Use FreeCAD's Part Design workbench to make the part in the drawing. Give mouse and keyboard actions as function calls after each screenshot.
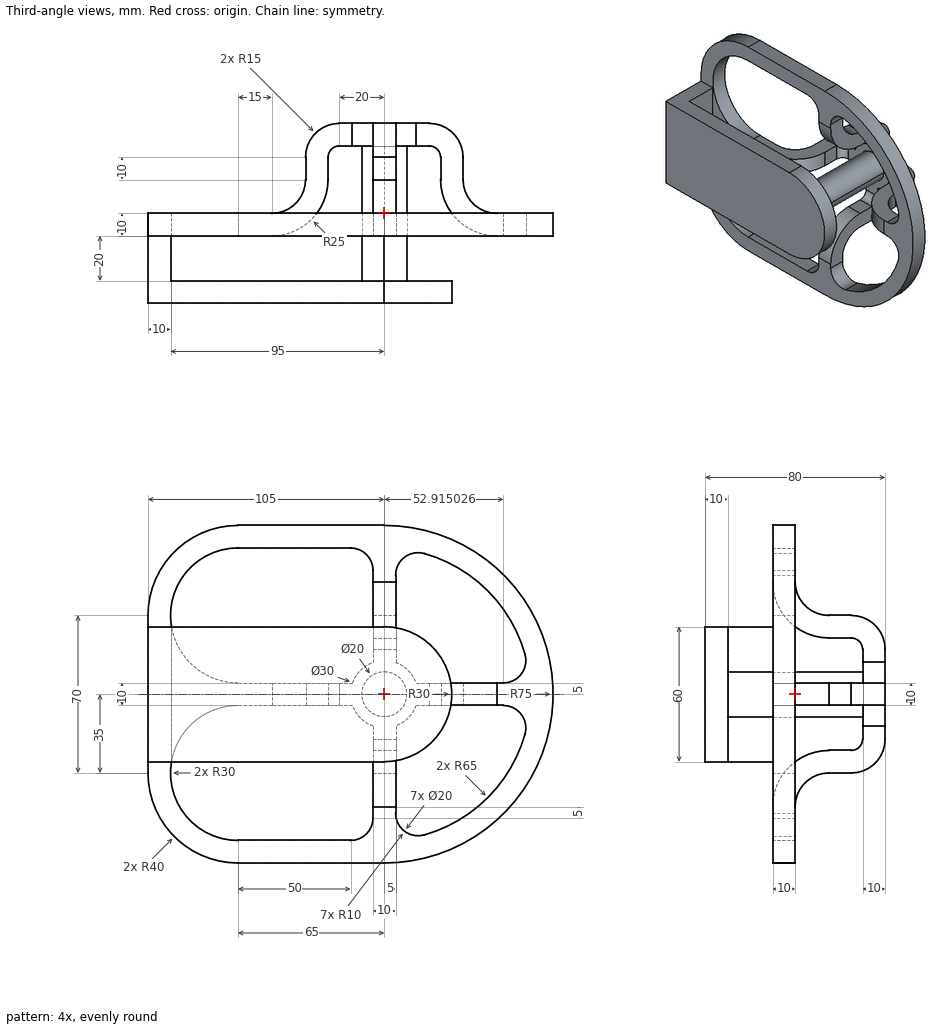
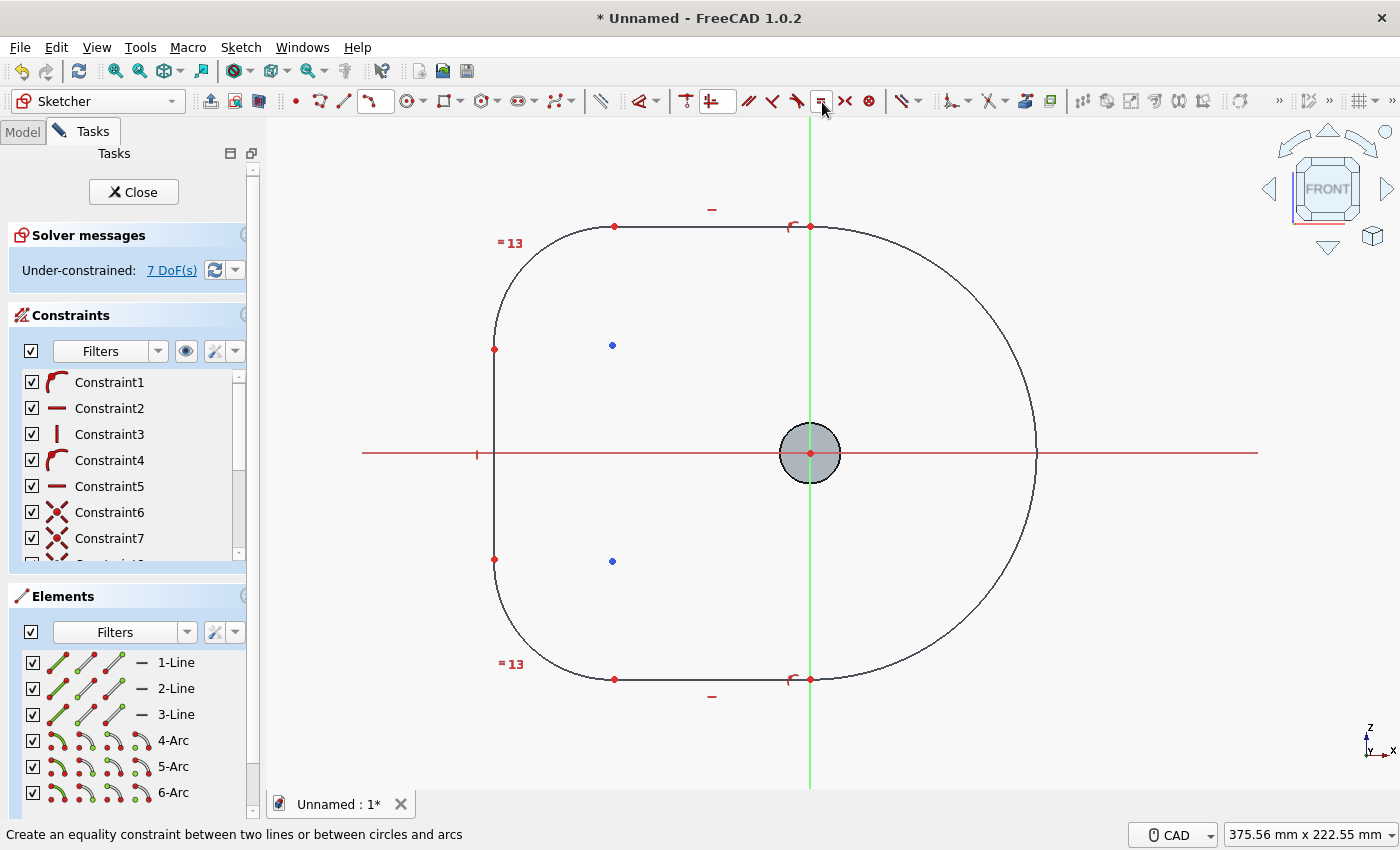
click(507, 615)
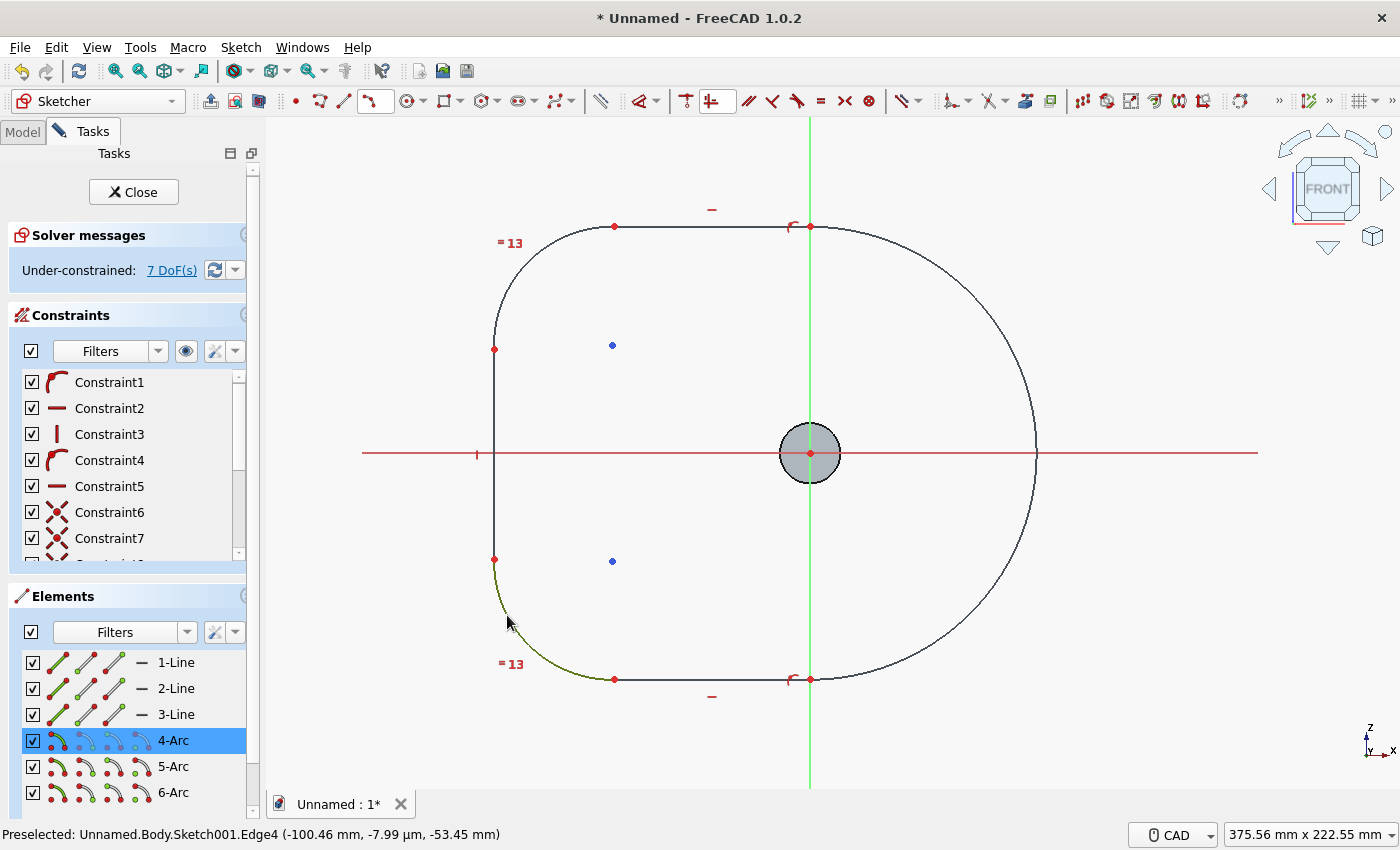
key(k)
key(r)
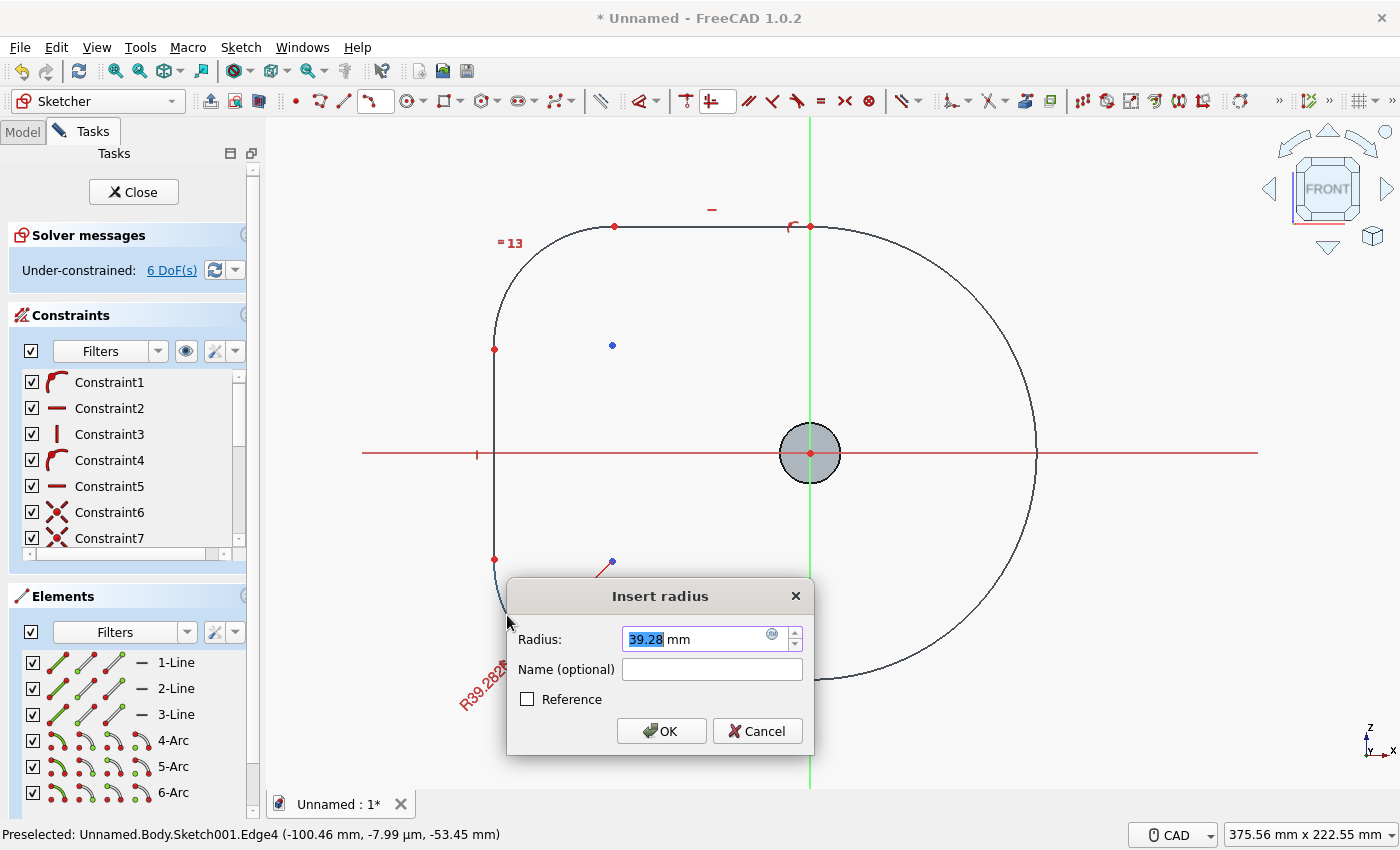
text(40)
key(Return)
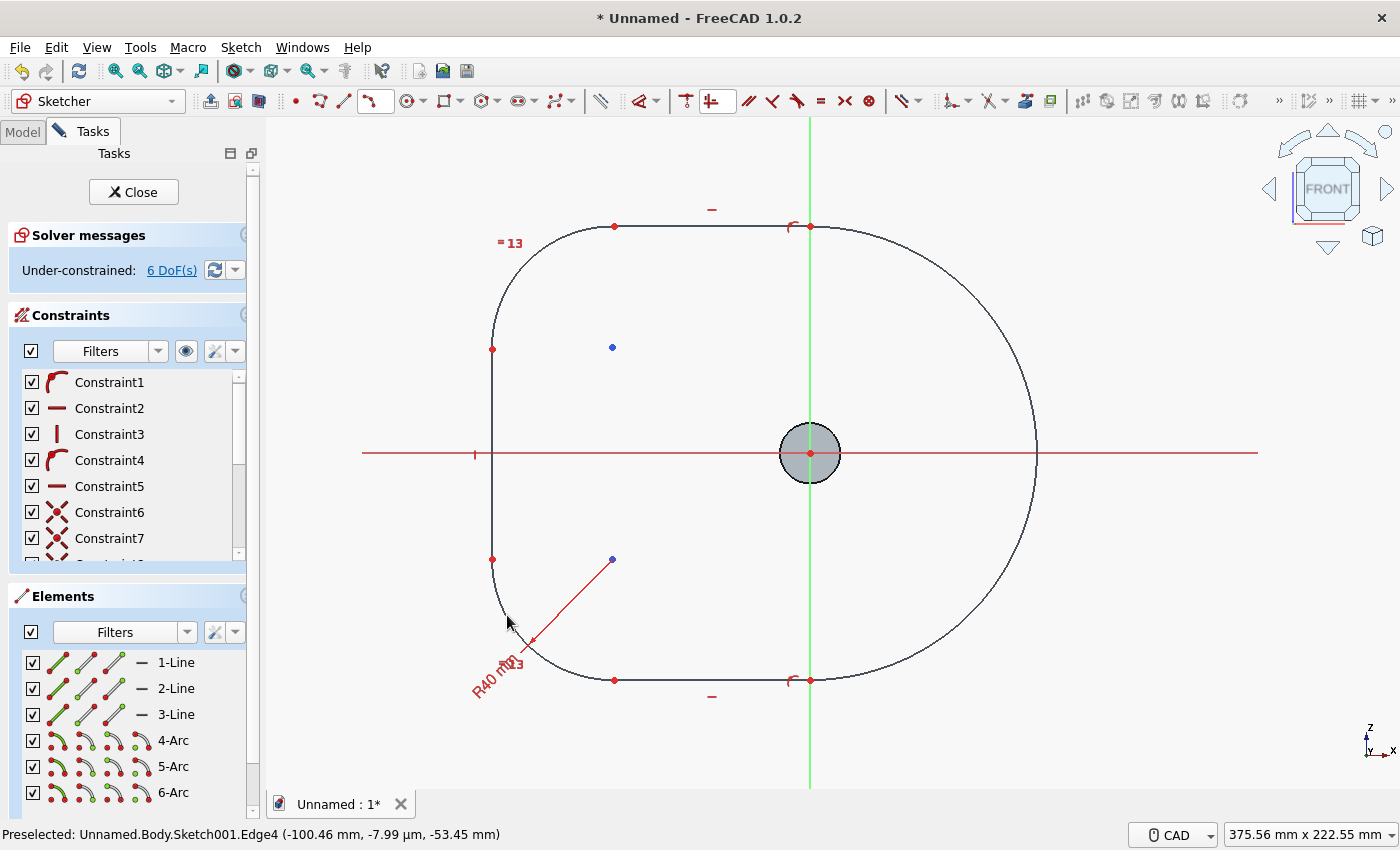
click(994, 587)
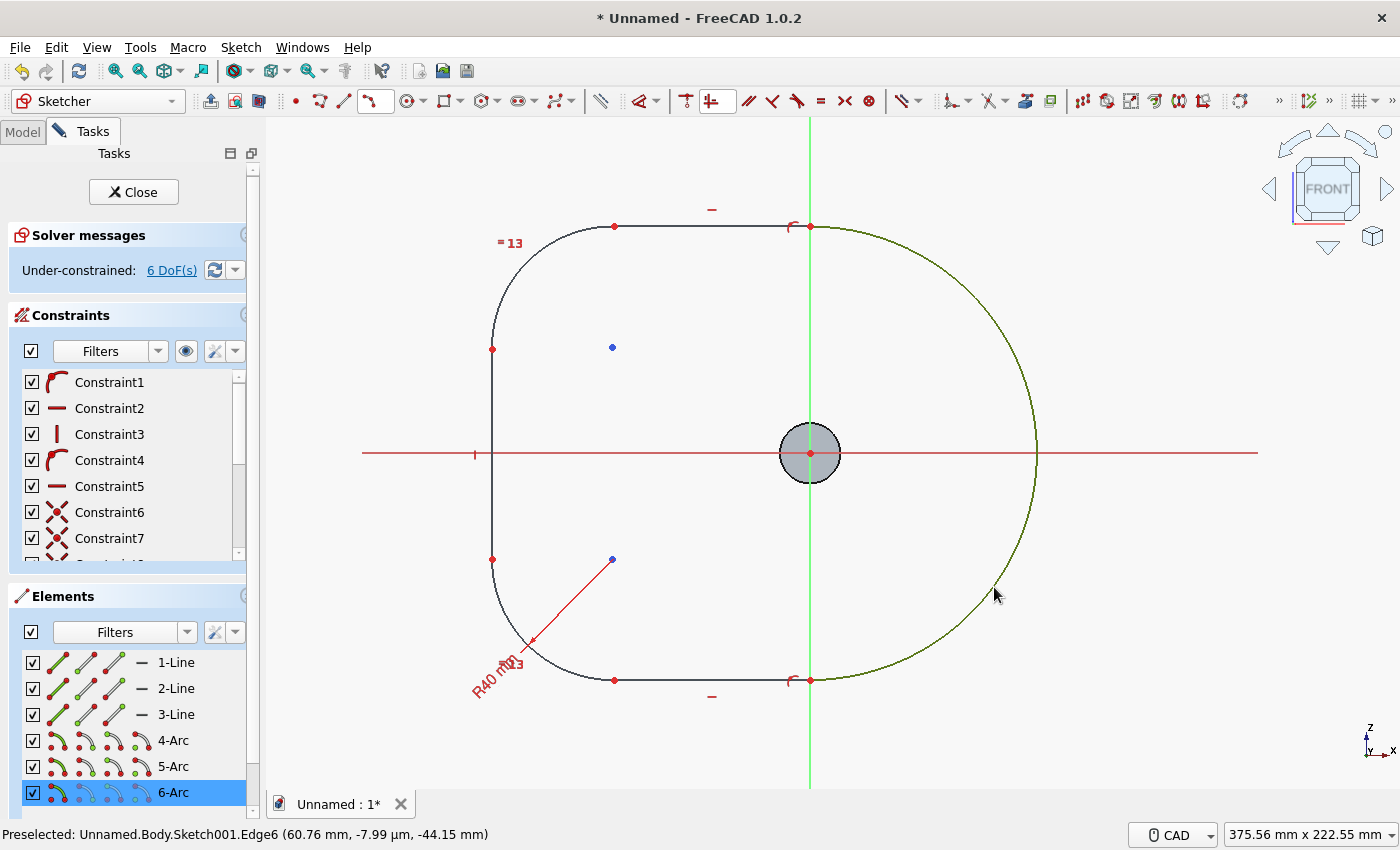
key(k)
key(r)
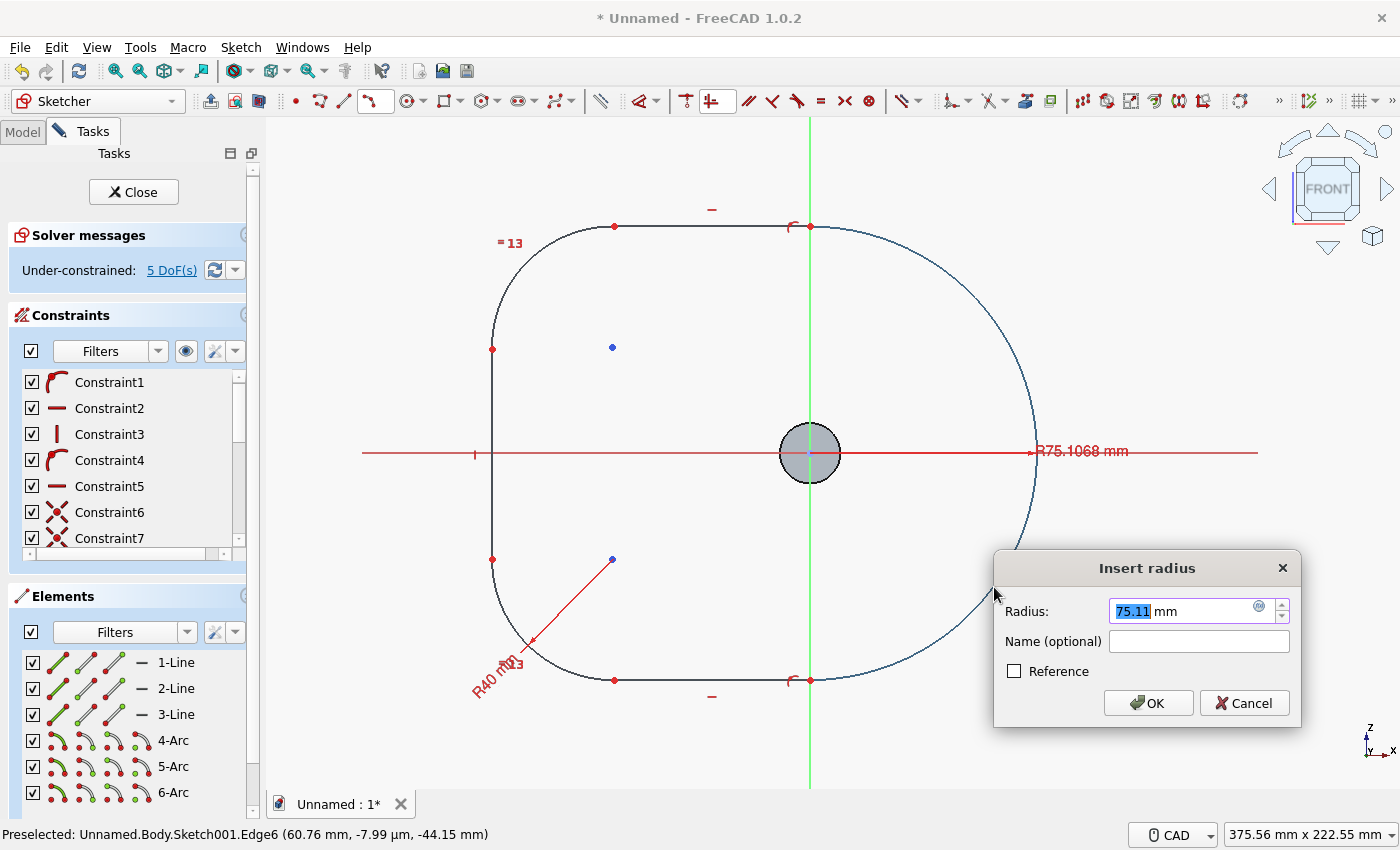
text(75)
key(Return)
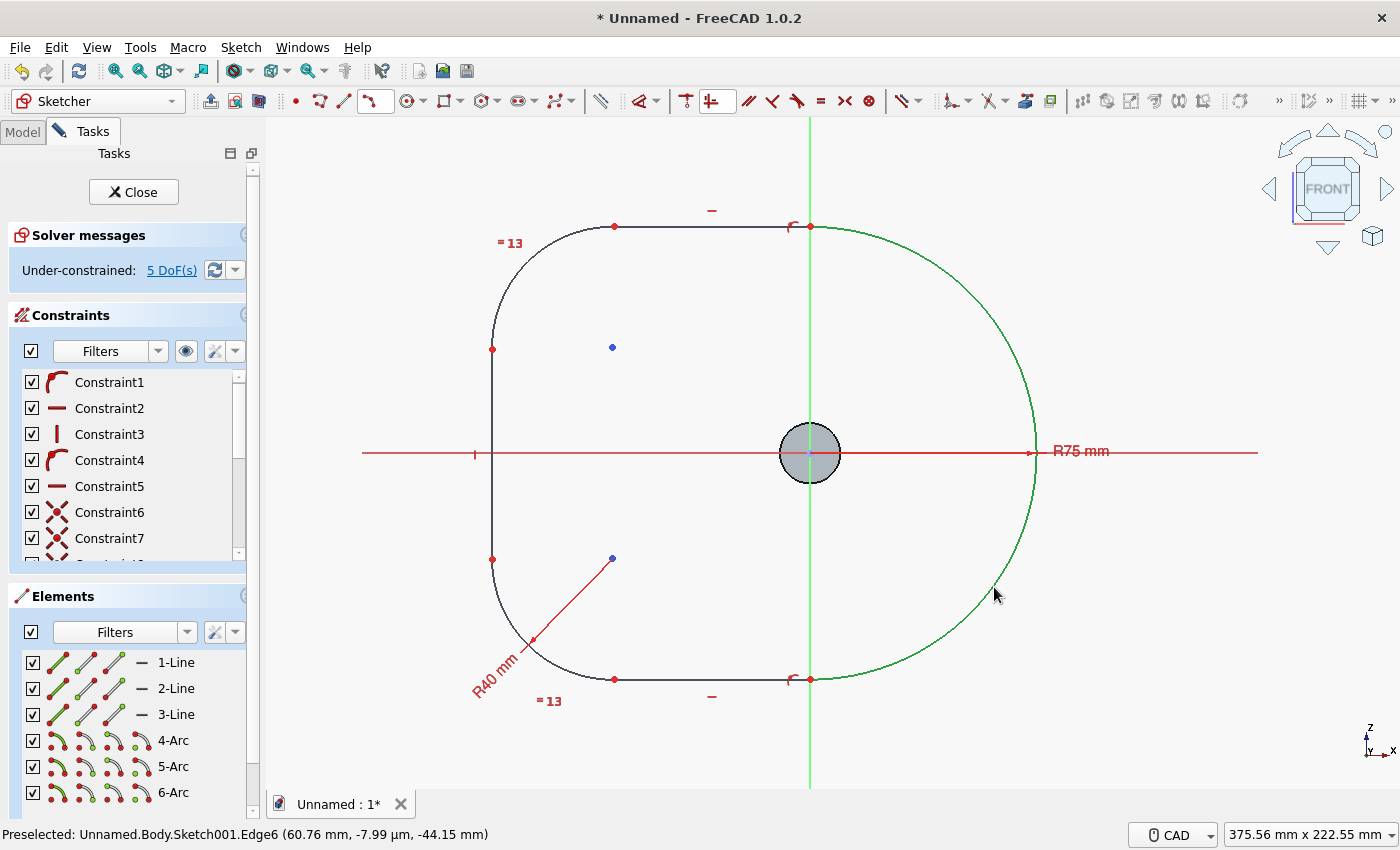
click(751, 680)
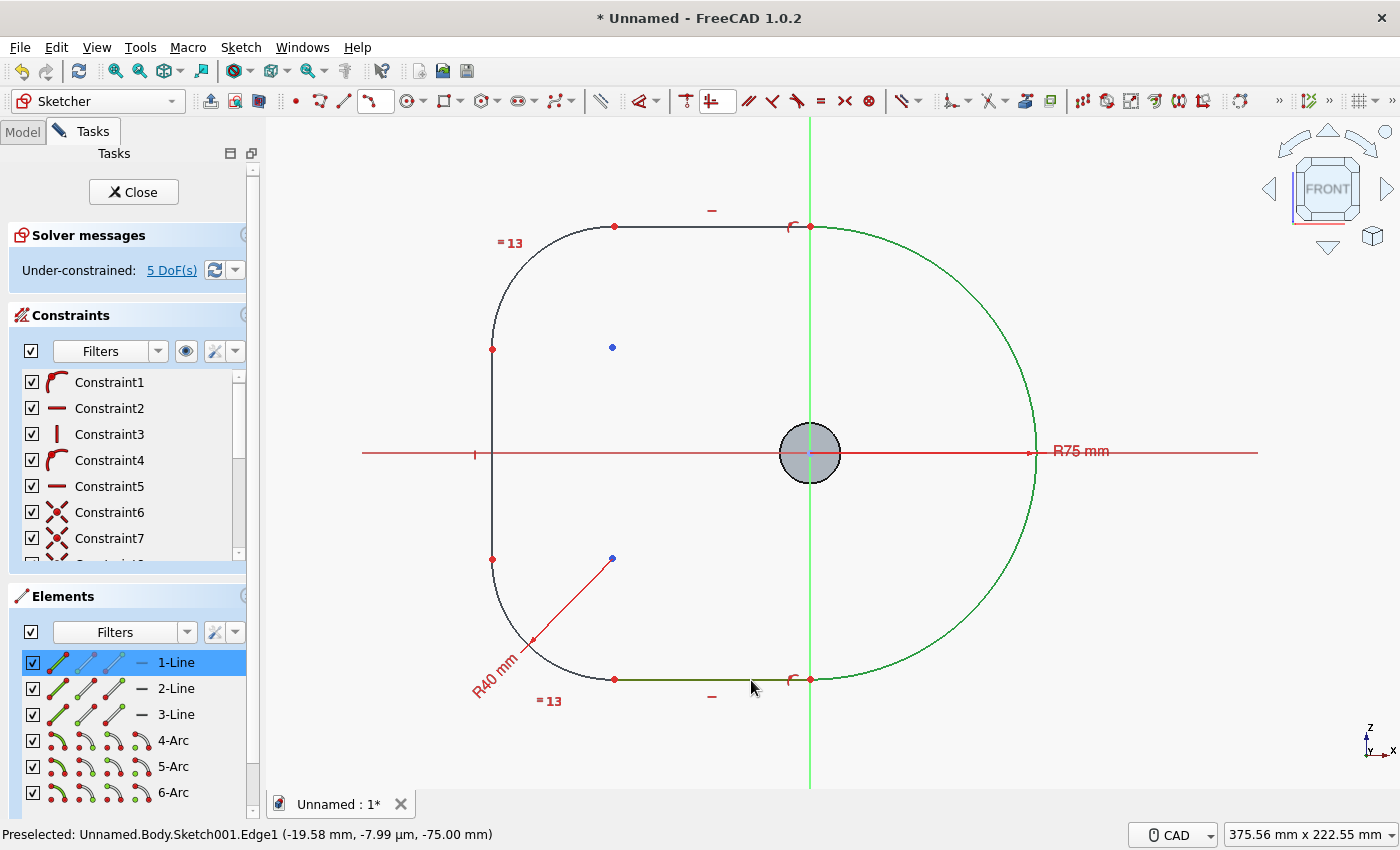
click(658, 102)